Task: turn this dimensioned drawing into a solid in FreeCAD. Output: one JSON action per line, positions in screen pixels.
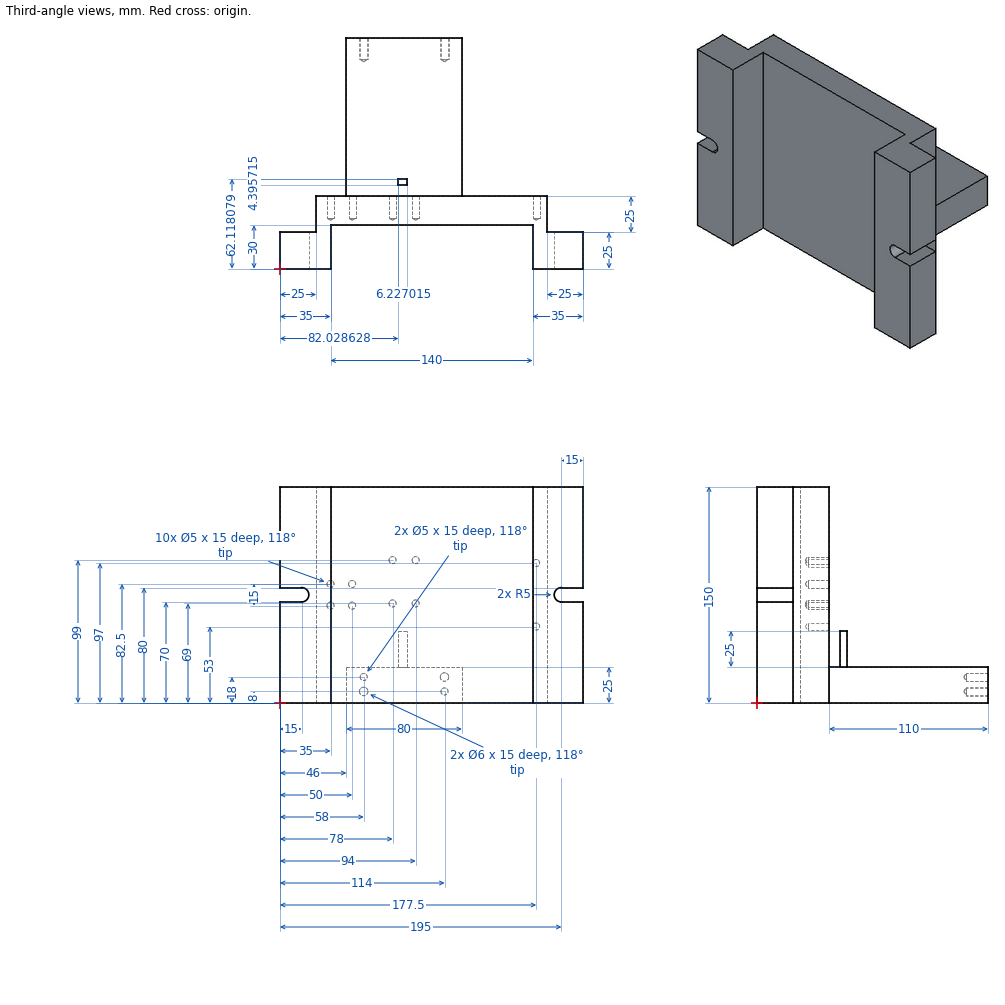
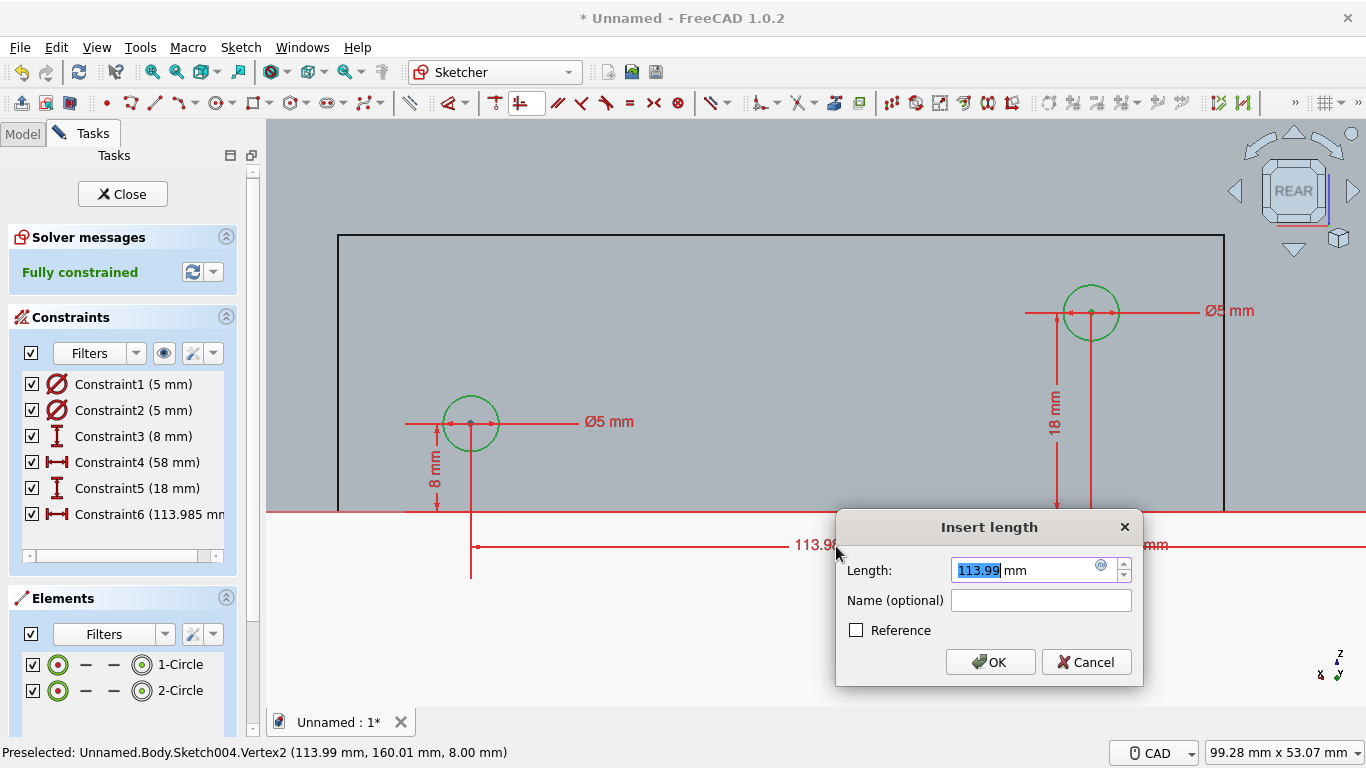
{"action": "type", "text": "114"}
{"action": "key", "text": "Return"}
{"action": "key", "text": "Escape"}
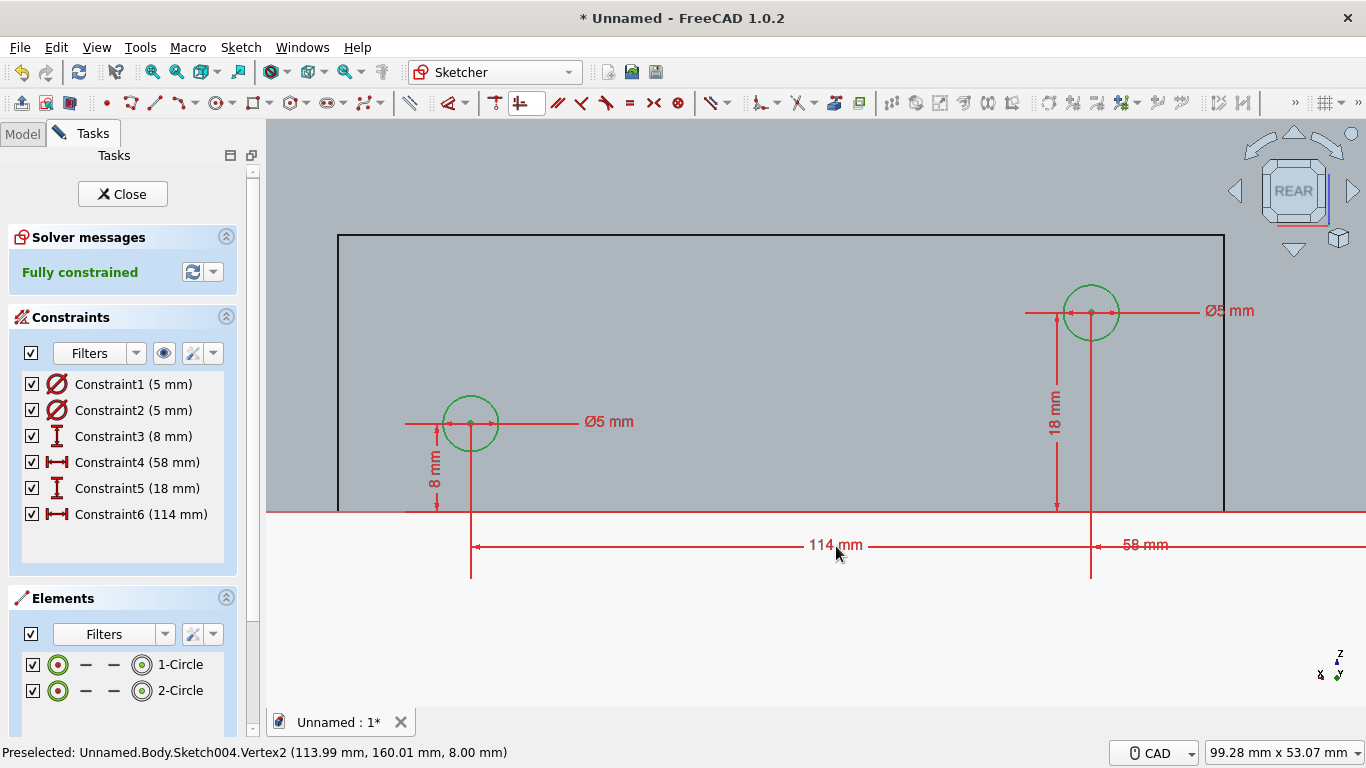
{"action": "left_click", "coordinate": [123, 194]}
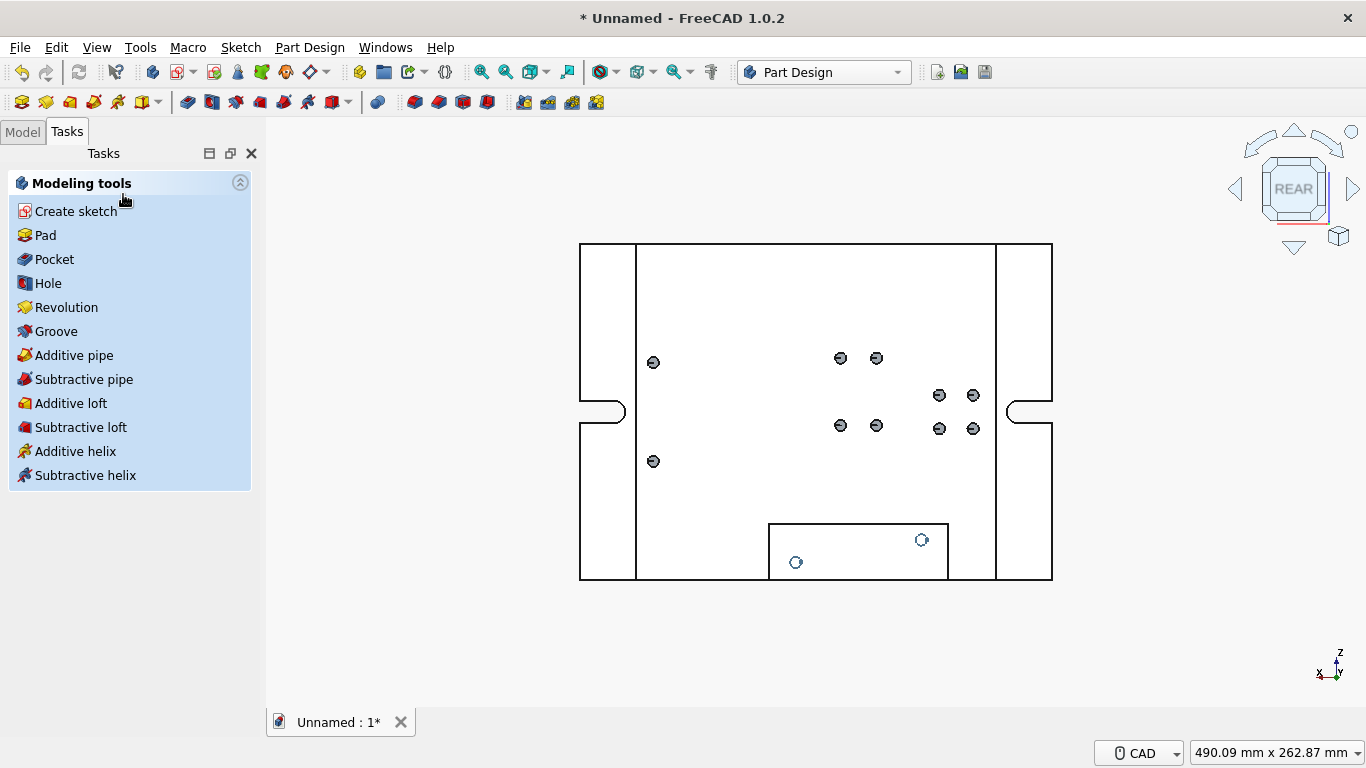
{"action": "left_click", "coordinate": [212, 102]}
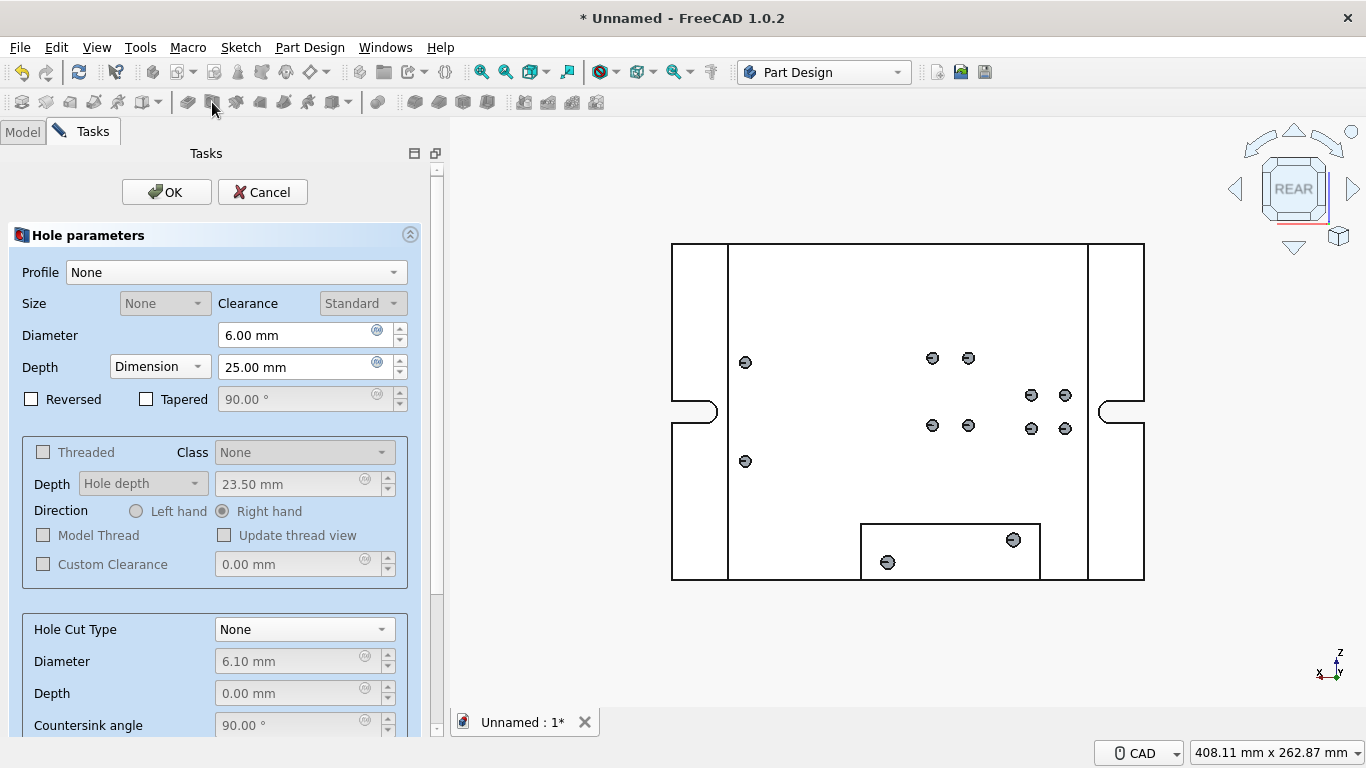
{"action": "triple_click", "coordinate": [305, 335]}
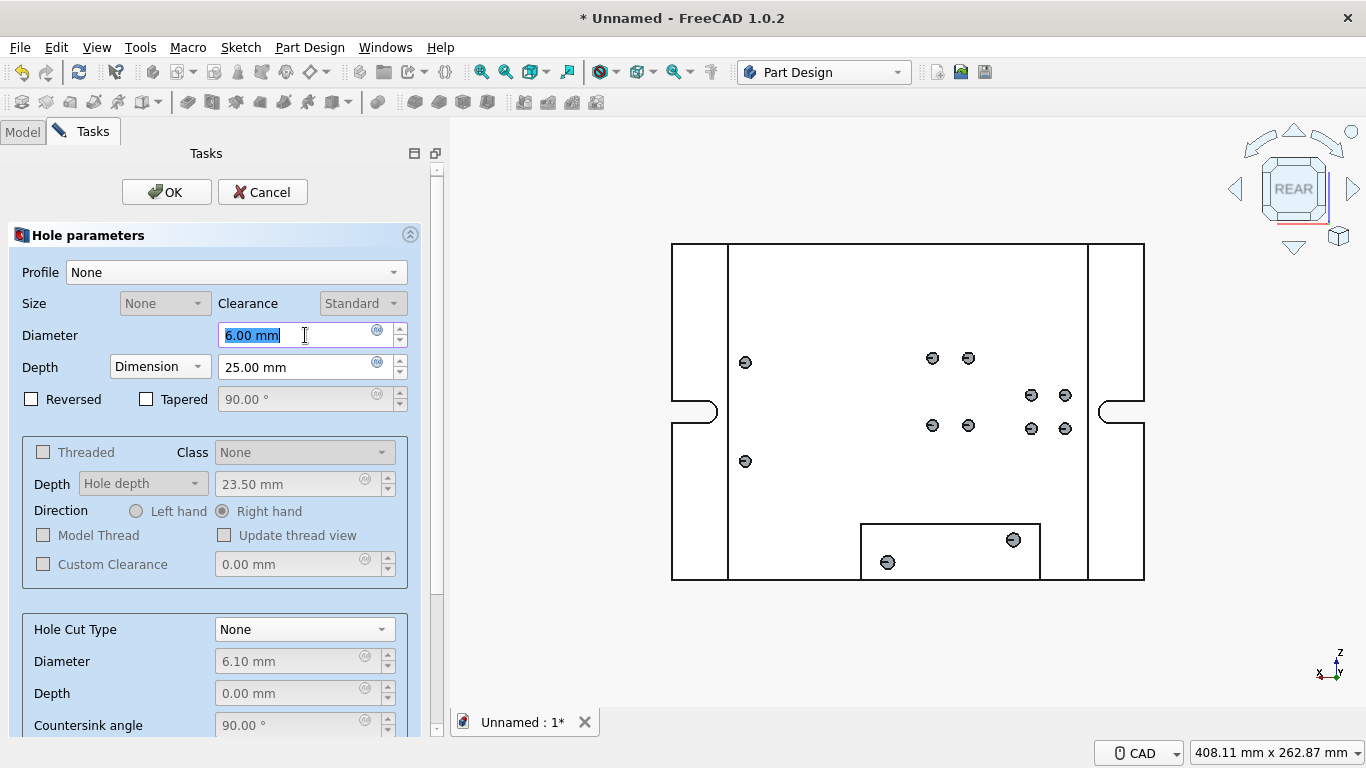
{"action": "type", "text": "5"}
{"action": "key", "text": "Tab"}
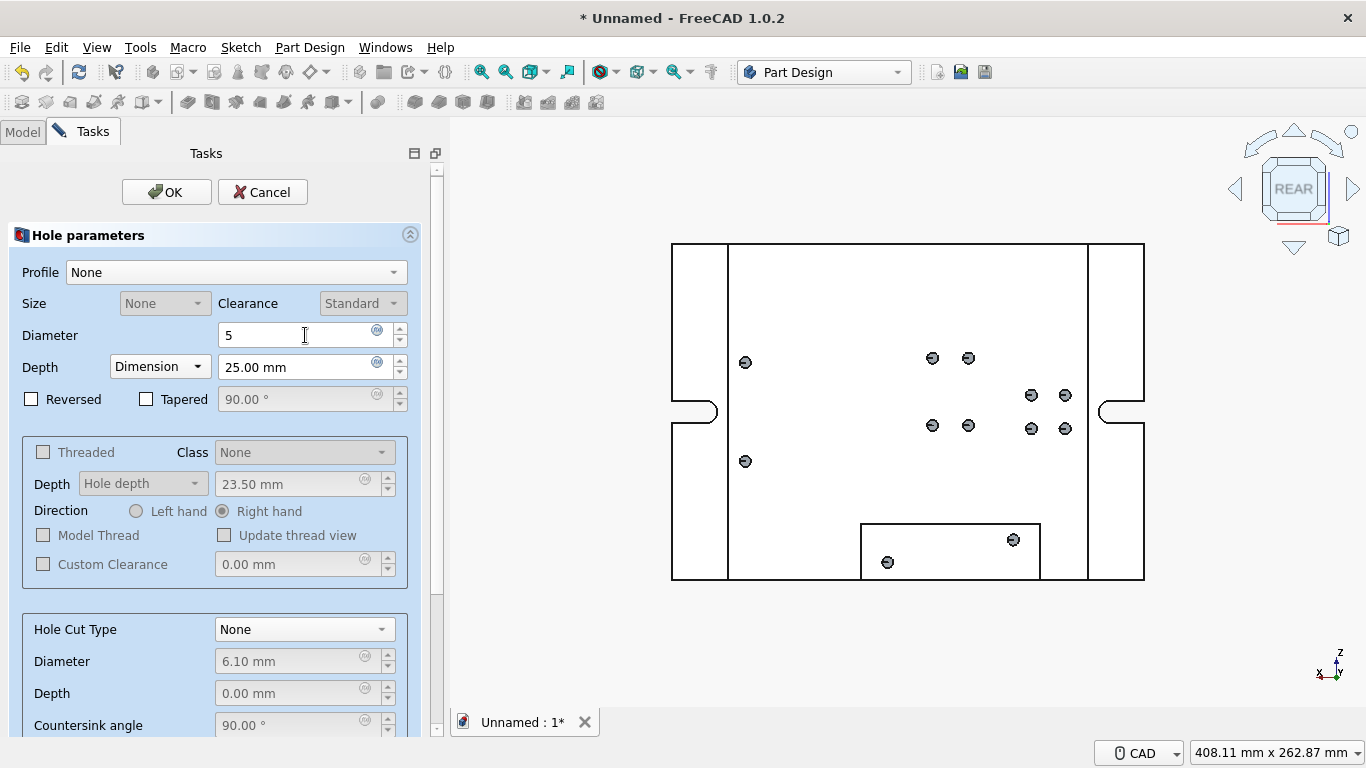
{"action": "triple_click", "coordinate": [305, 367]}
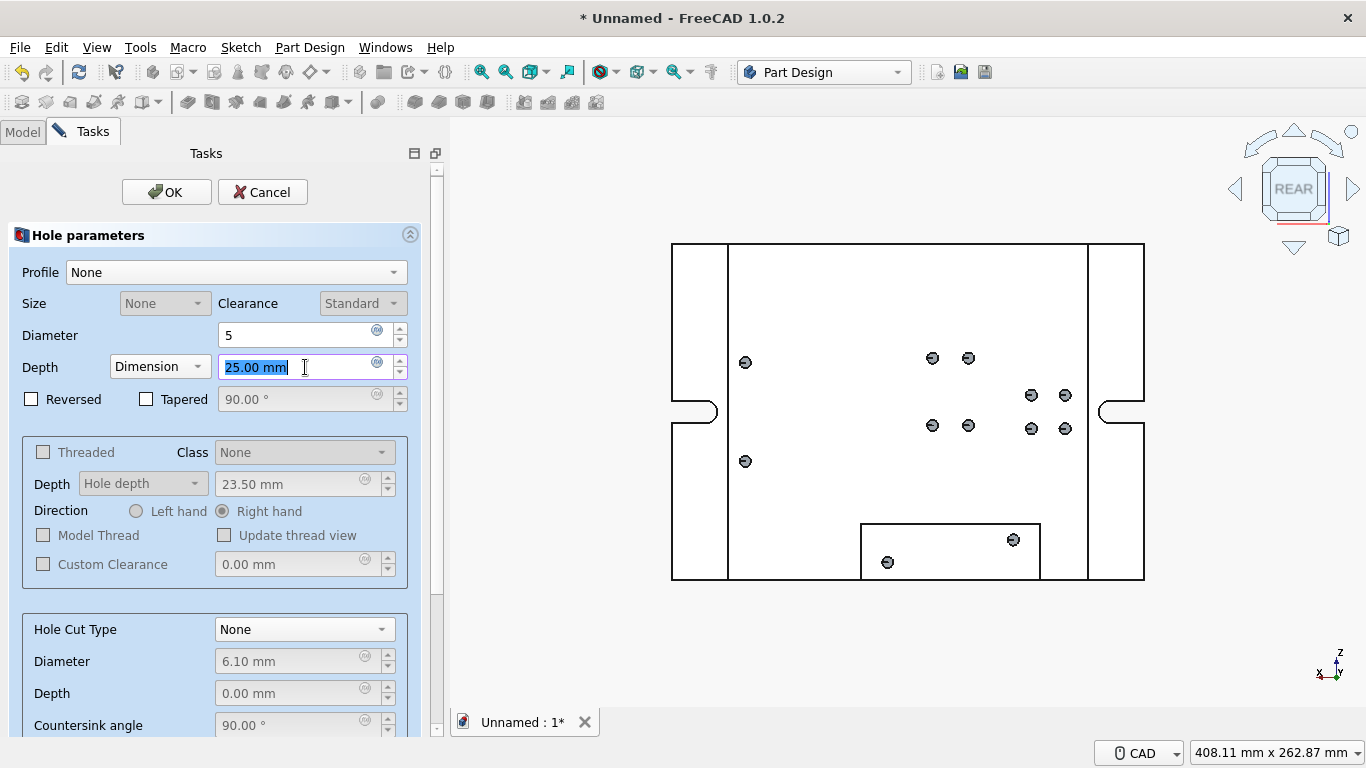
{"action": "type", "text": "15"}
{"action": "key", "text": "Tab"}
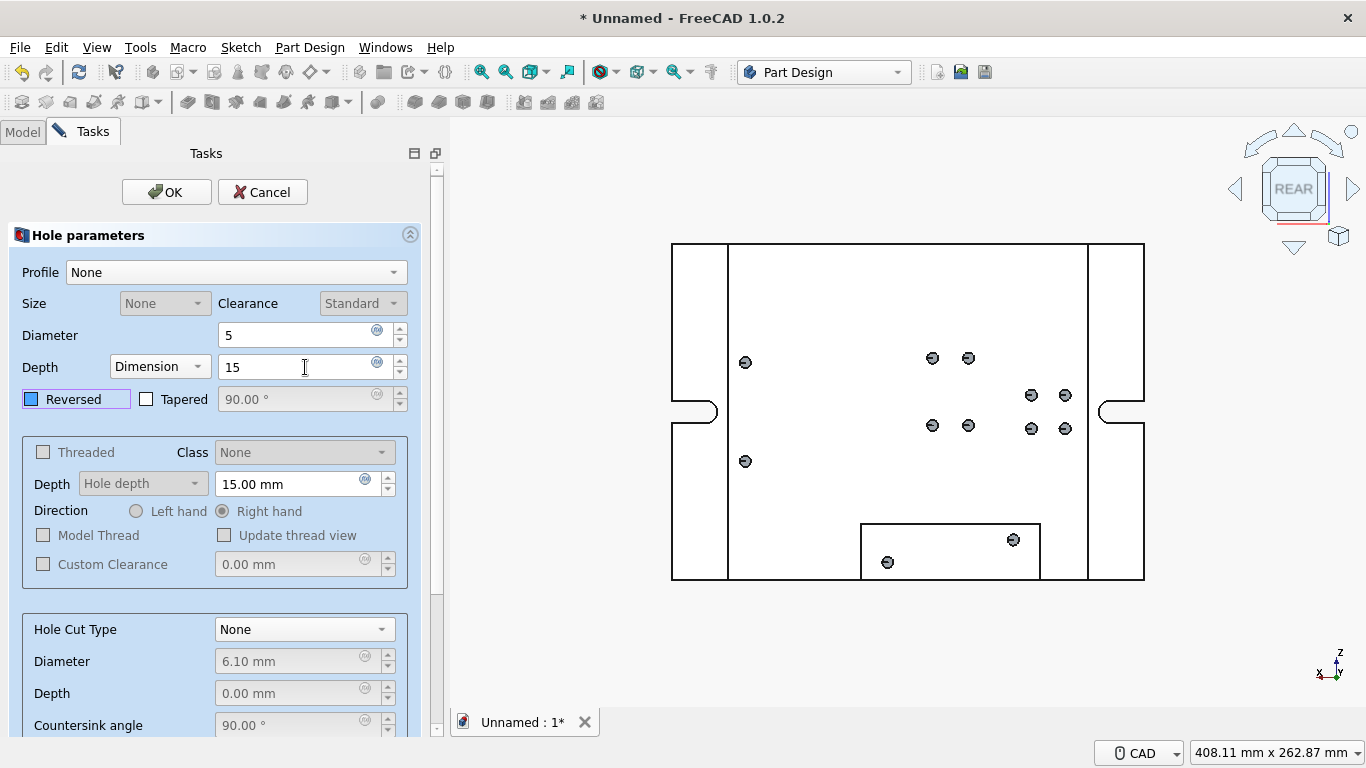
{"action": "left_click", "coordinate": [167, 192]}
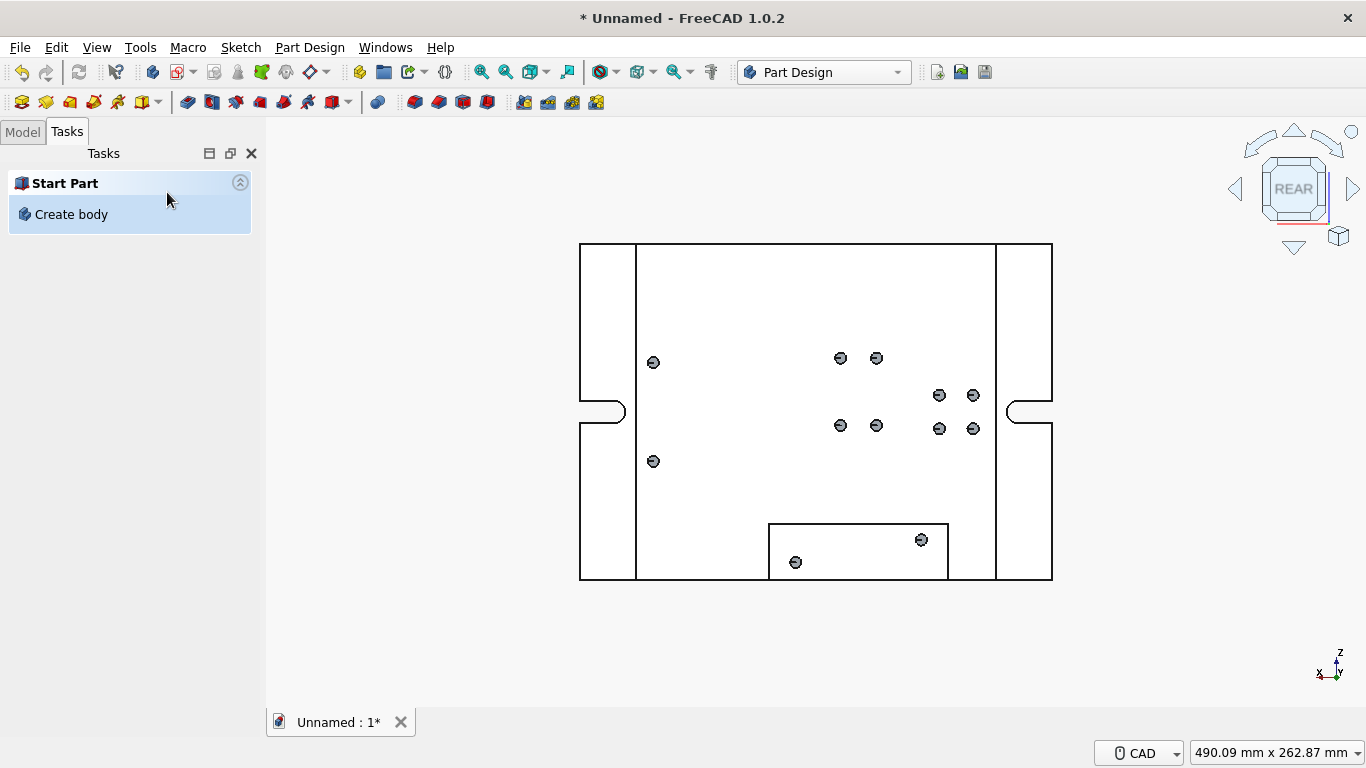
{"action": "left_click", "coordinate": [833, 551]}